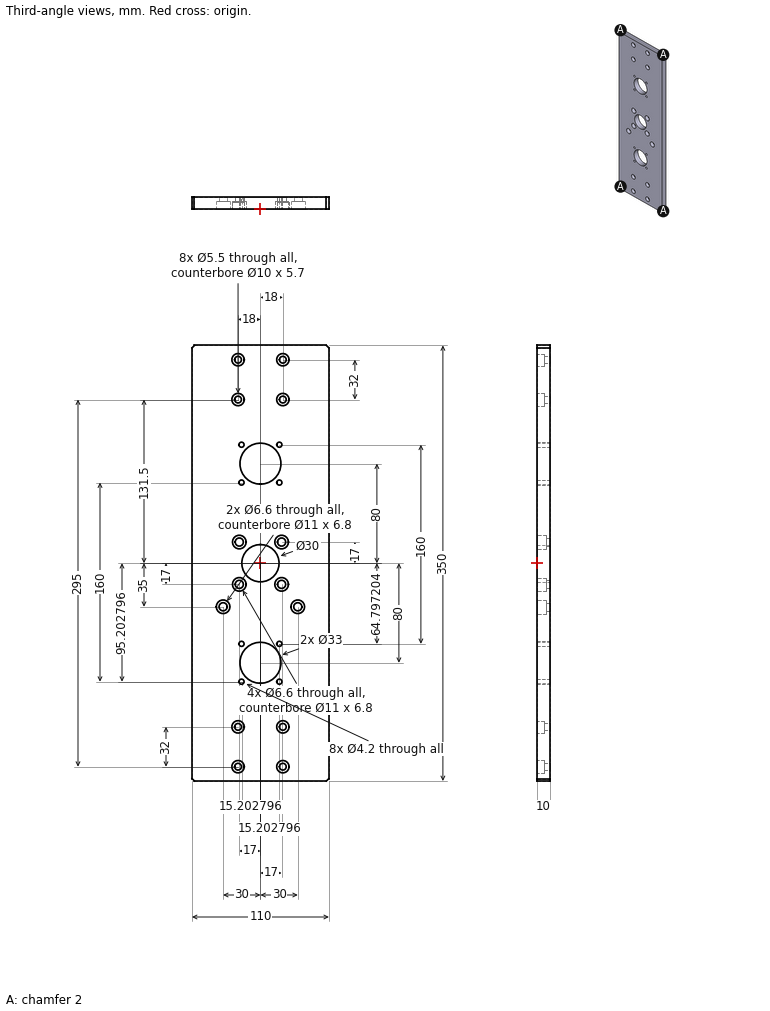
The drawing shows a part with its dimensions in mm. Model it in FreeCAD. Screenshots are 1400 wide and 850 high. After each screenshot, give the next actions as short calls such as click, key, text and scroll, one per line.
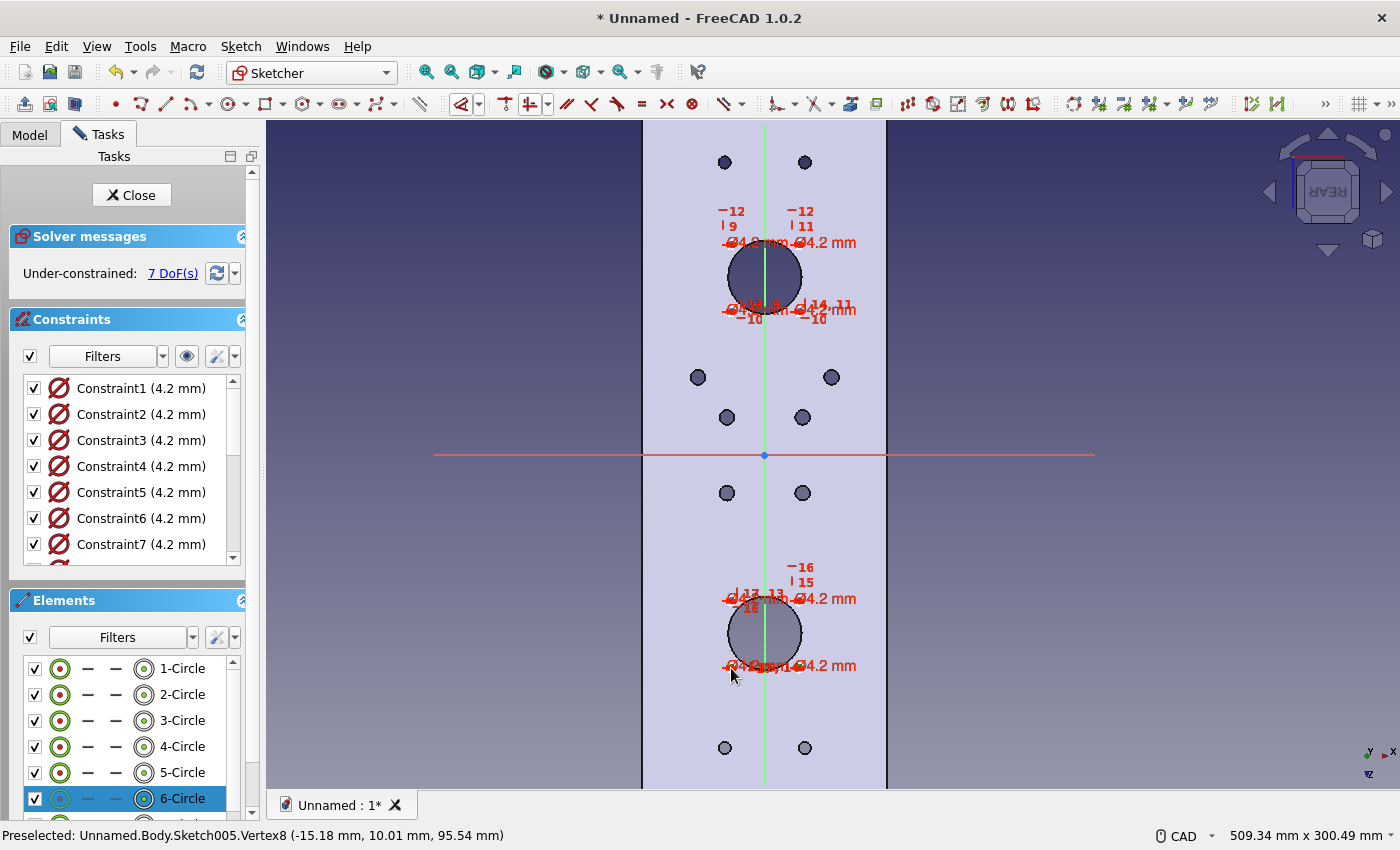
key(h)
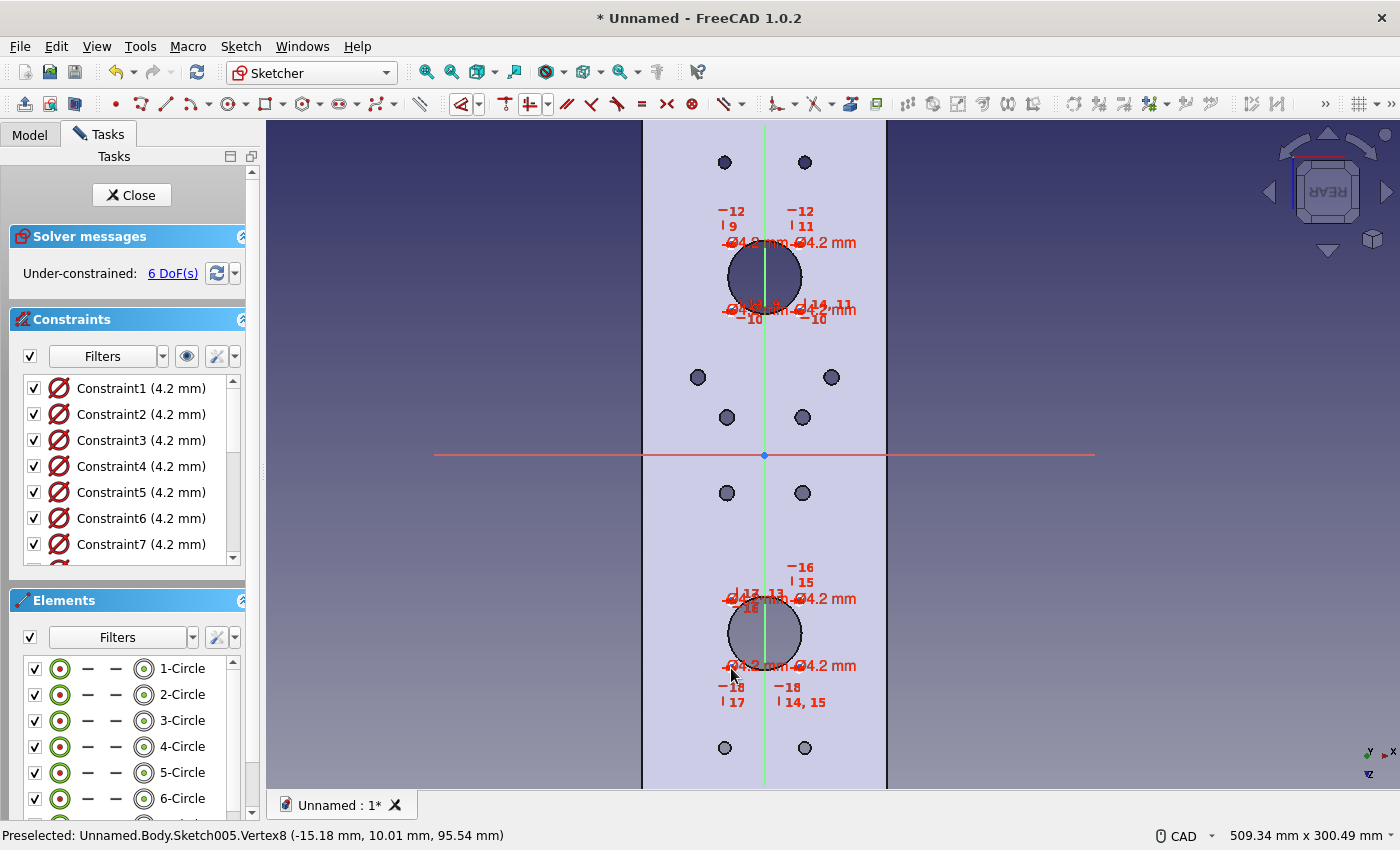
click(731, 245)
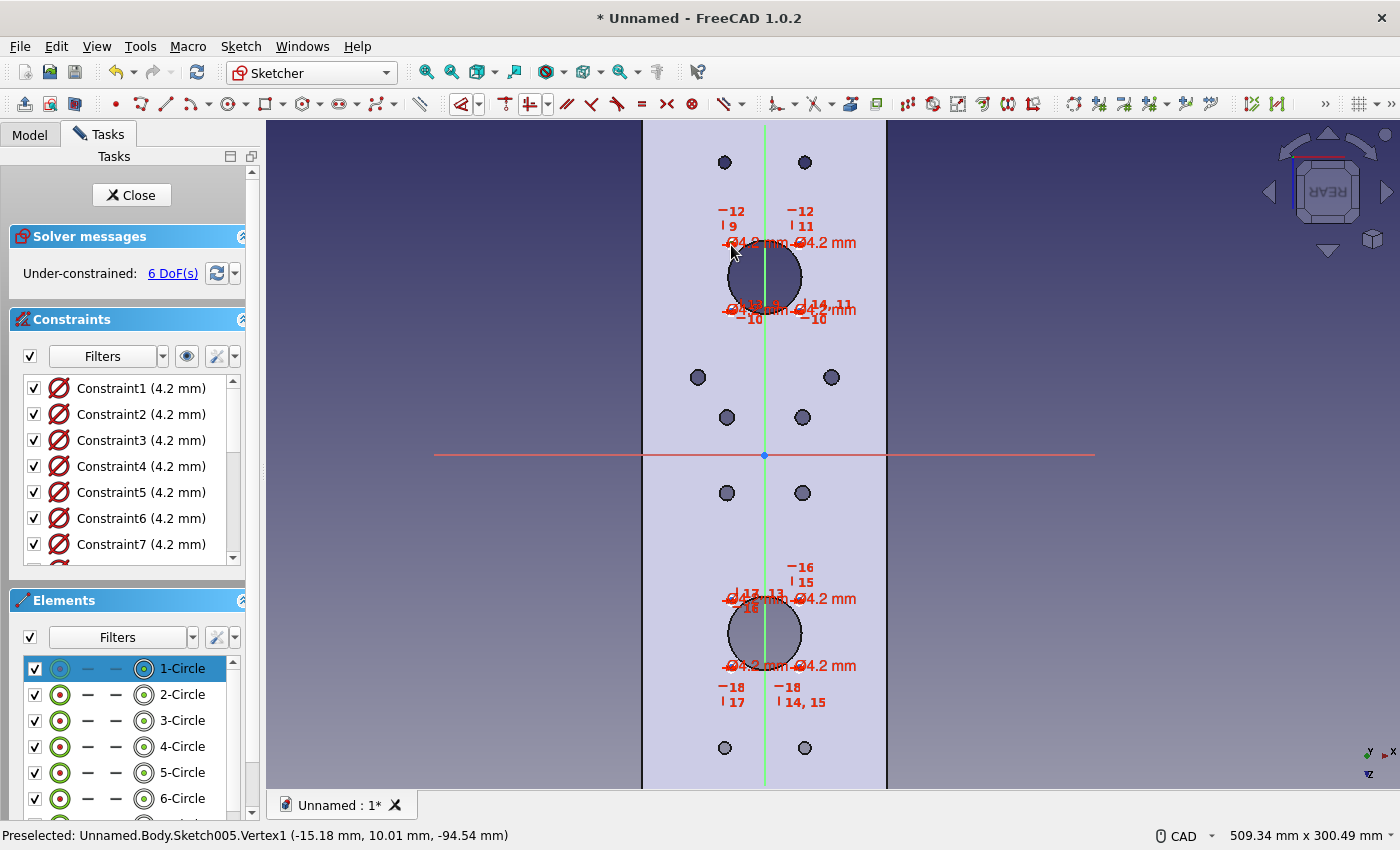
click(731, 601)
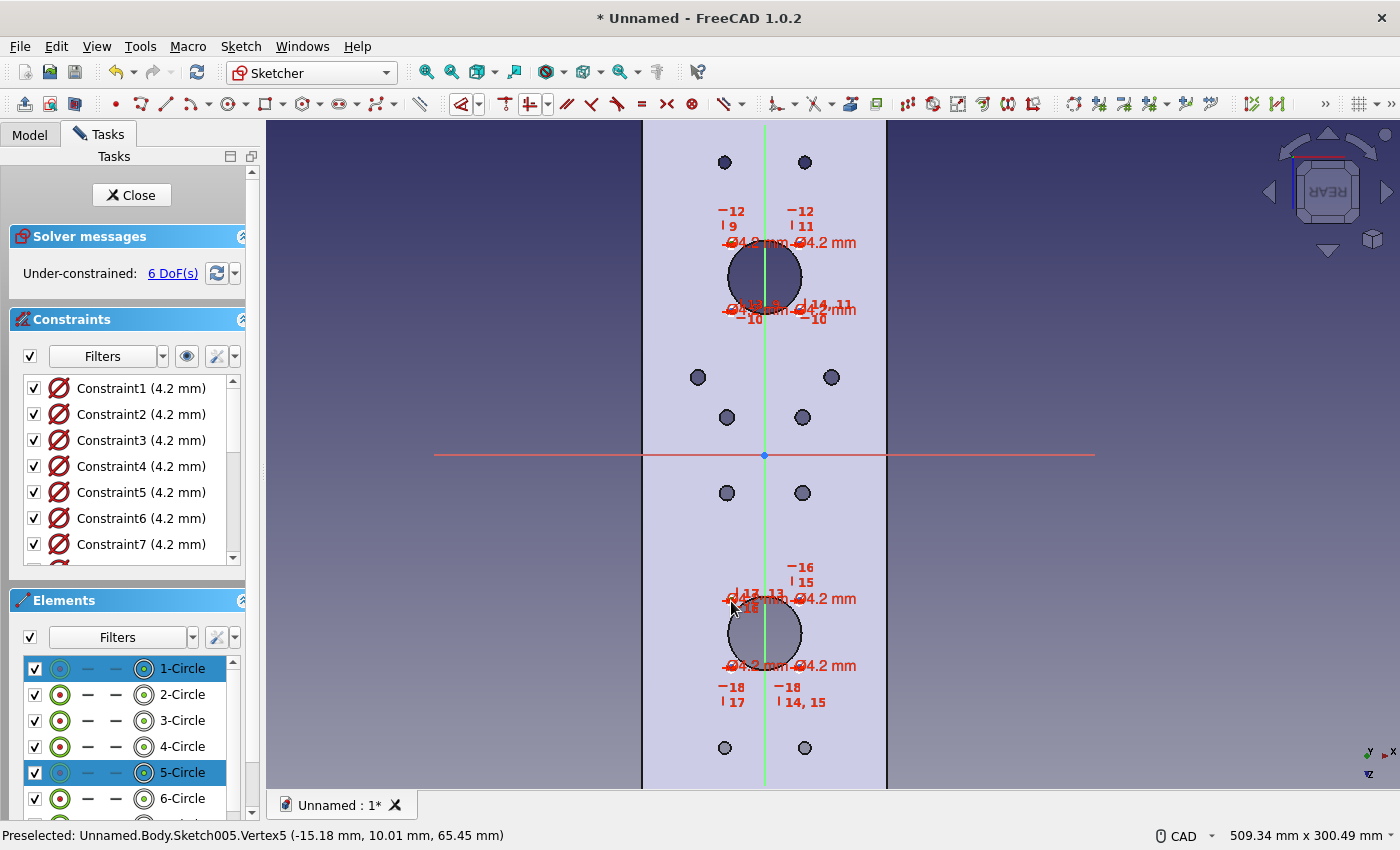
key(i)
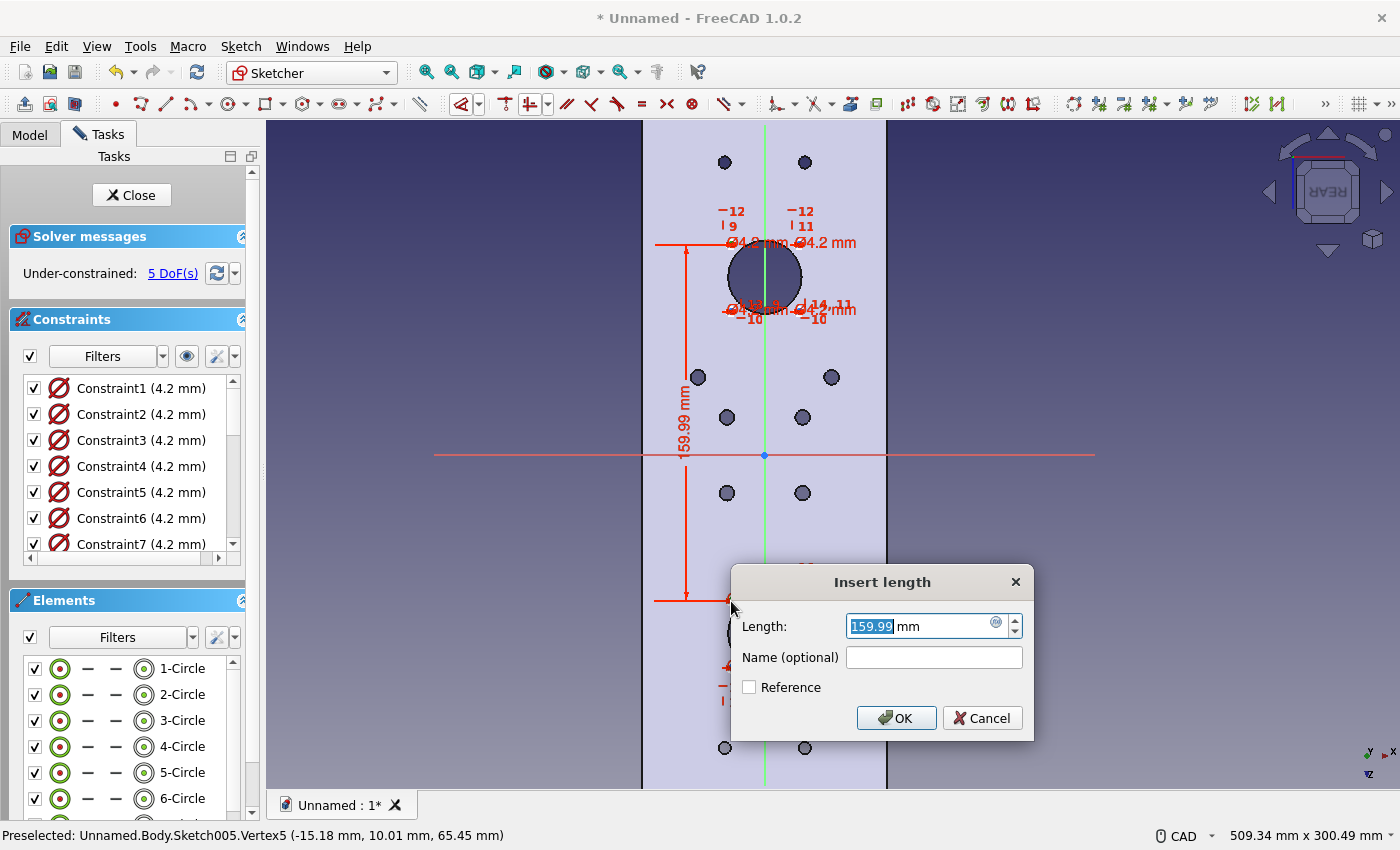
text(160)
key(Return)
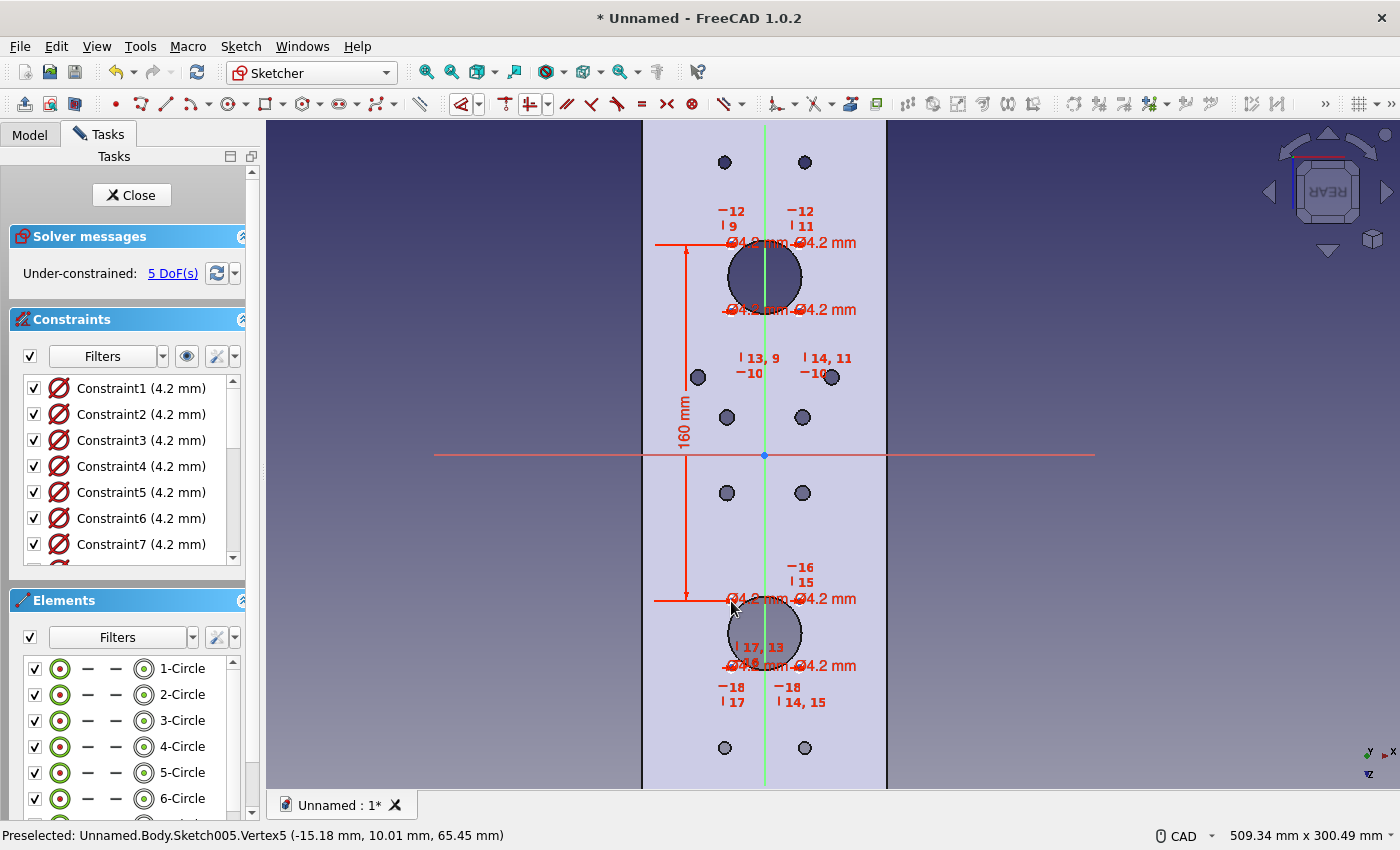
click(799, 312)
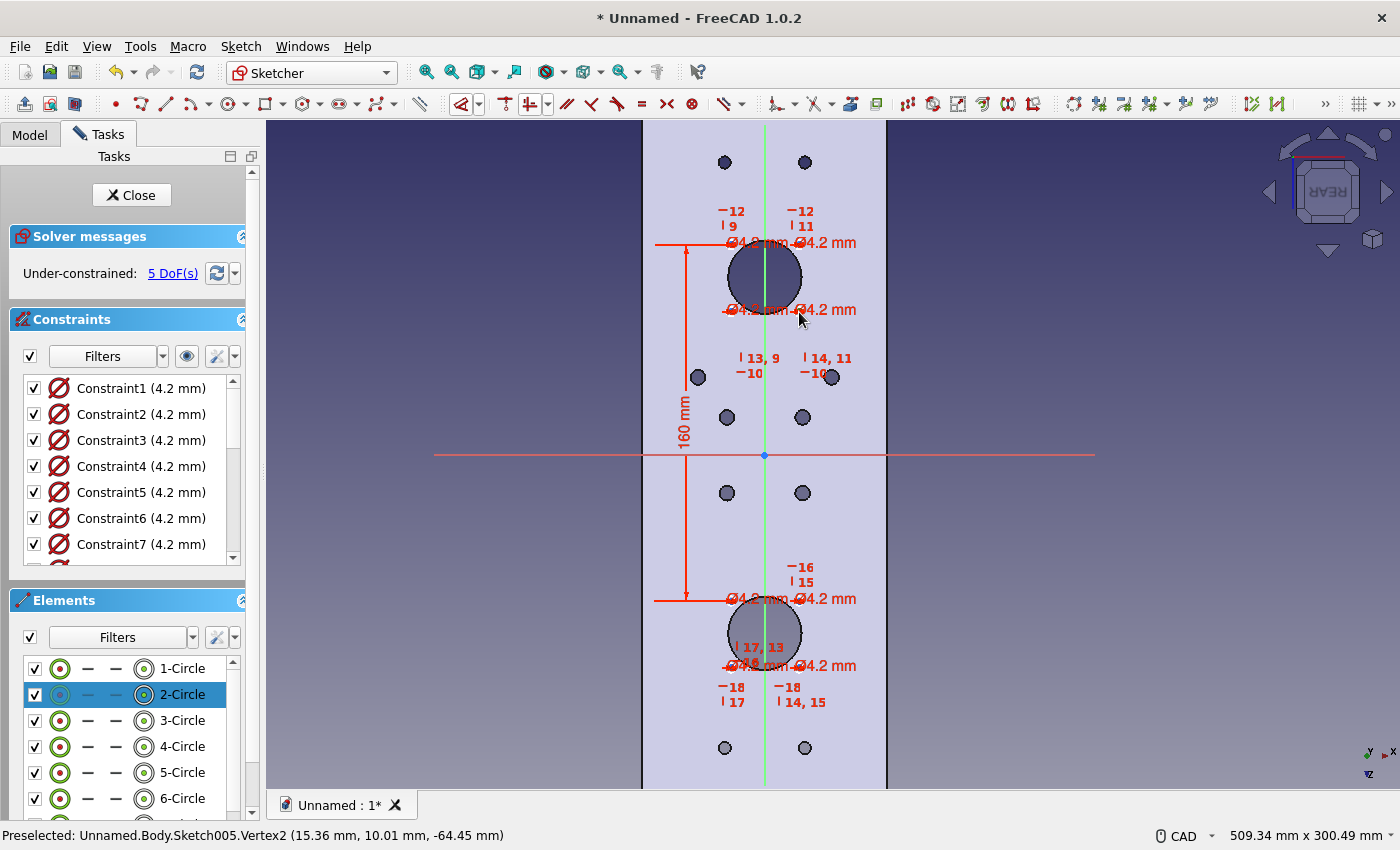
click(799, 668)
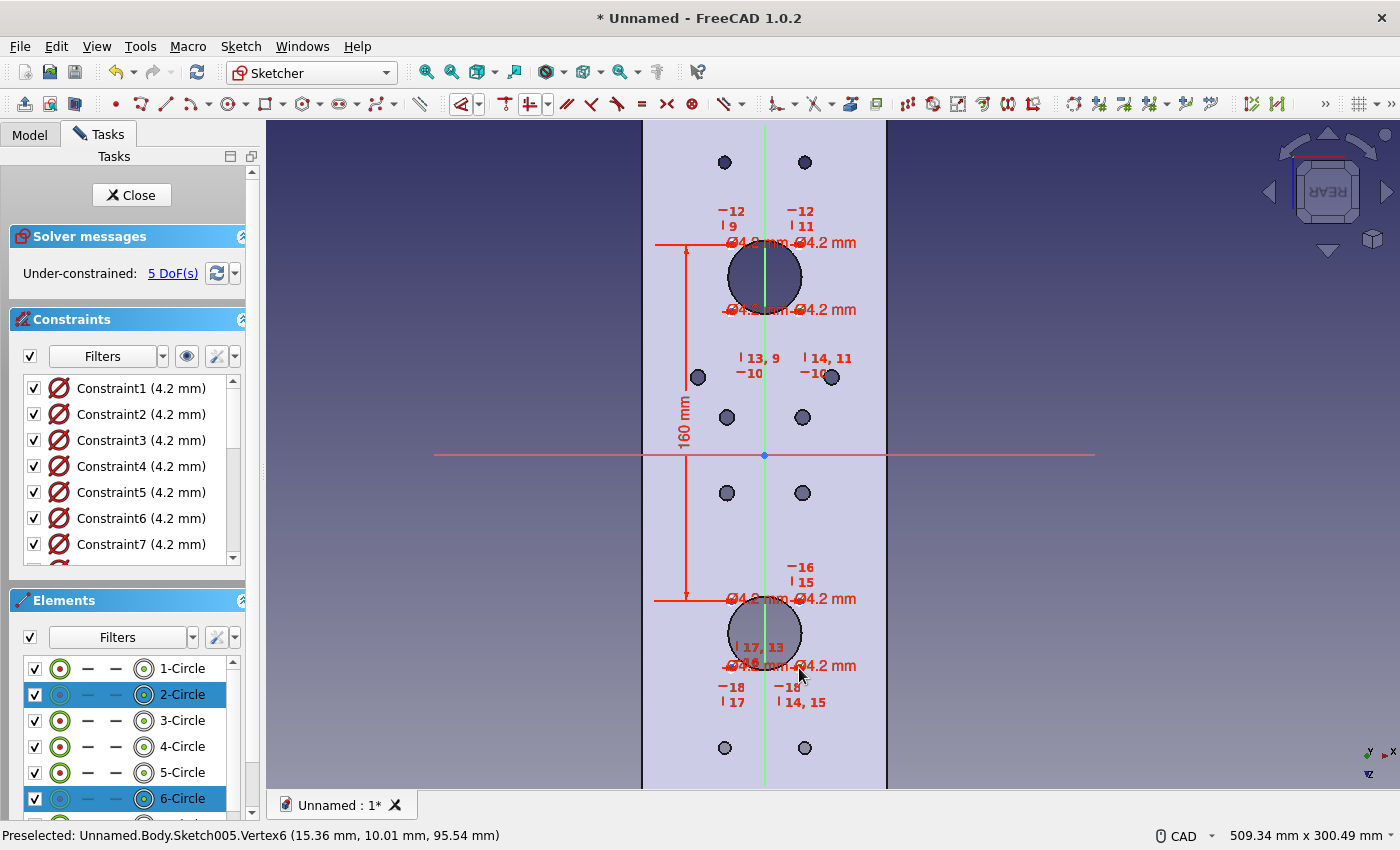
key(i)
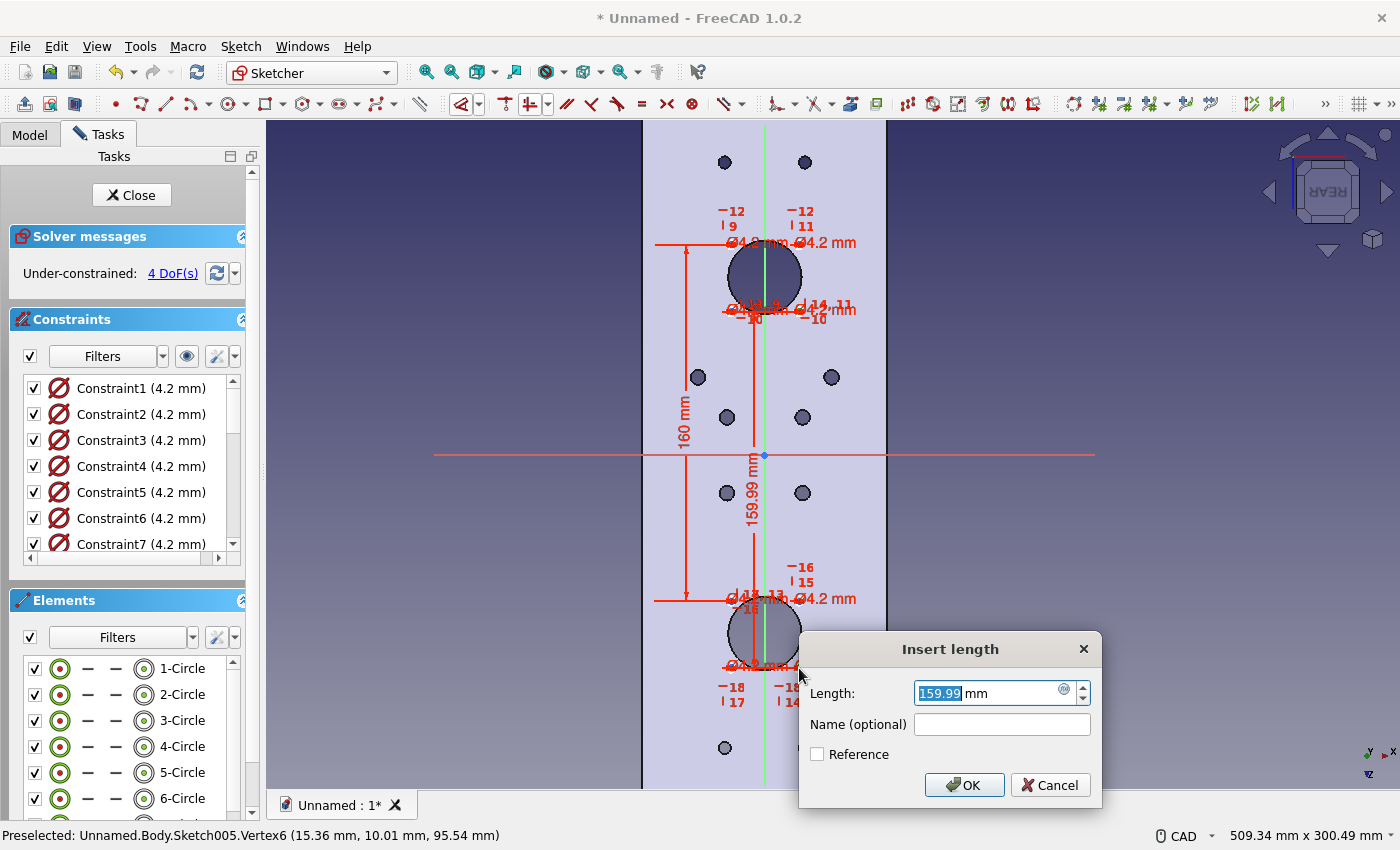
text(160)
key(Return)